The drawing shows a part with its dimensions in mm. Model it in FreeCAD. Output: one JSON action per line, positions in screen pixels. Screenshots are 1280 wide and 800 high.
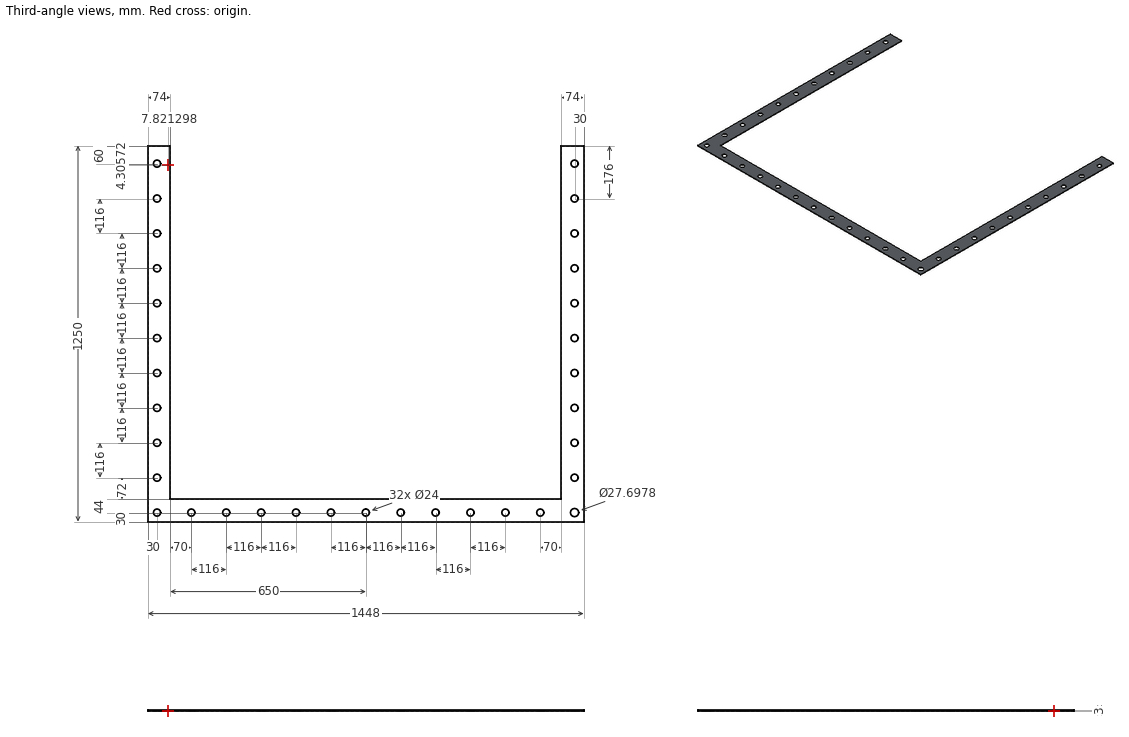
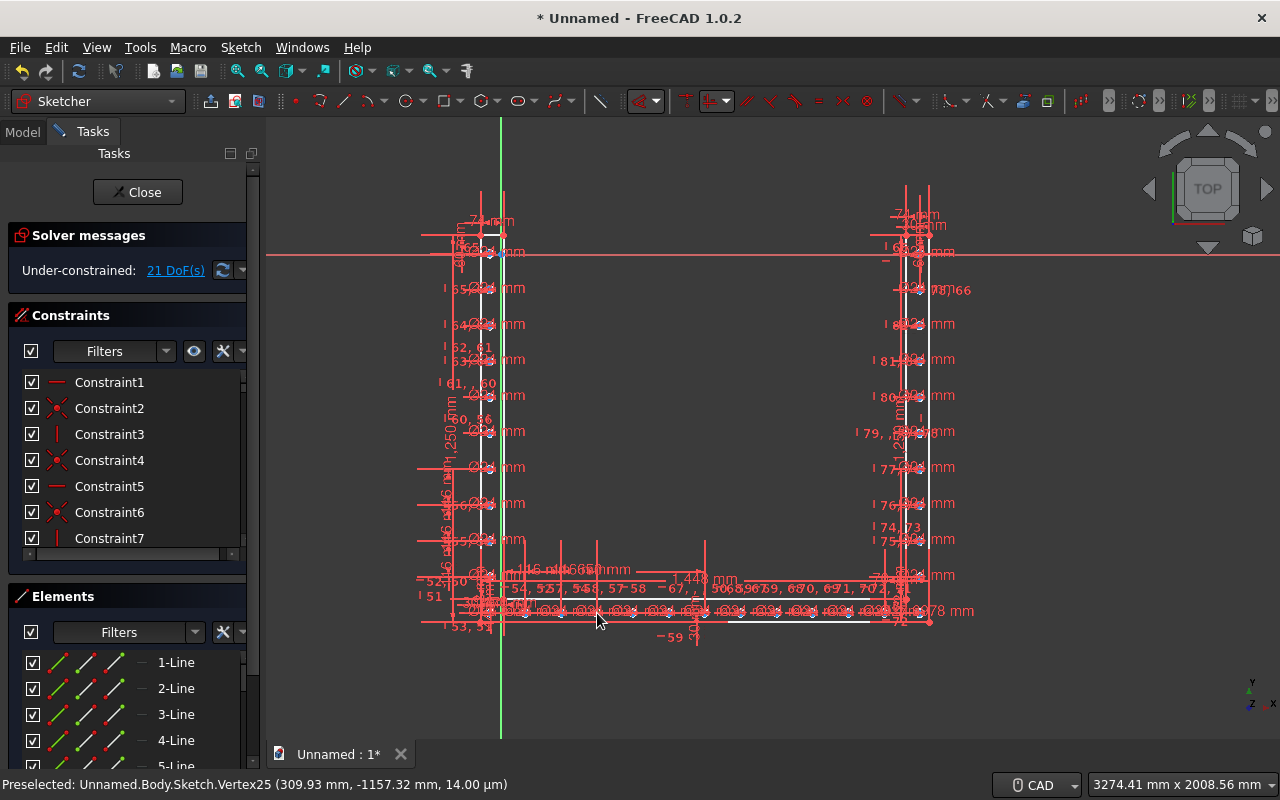
{"action": "left_click", "coordinate": [633, 613]}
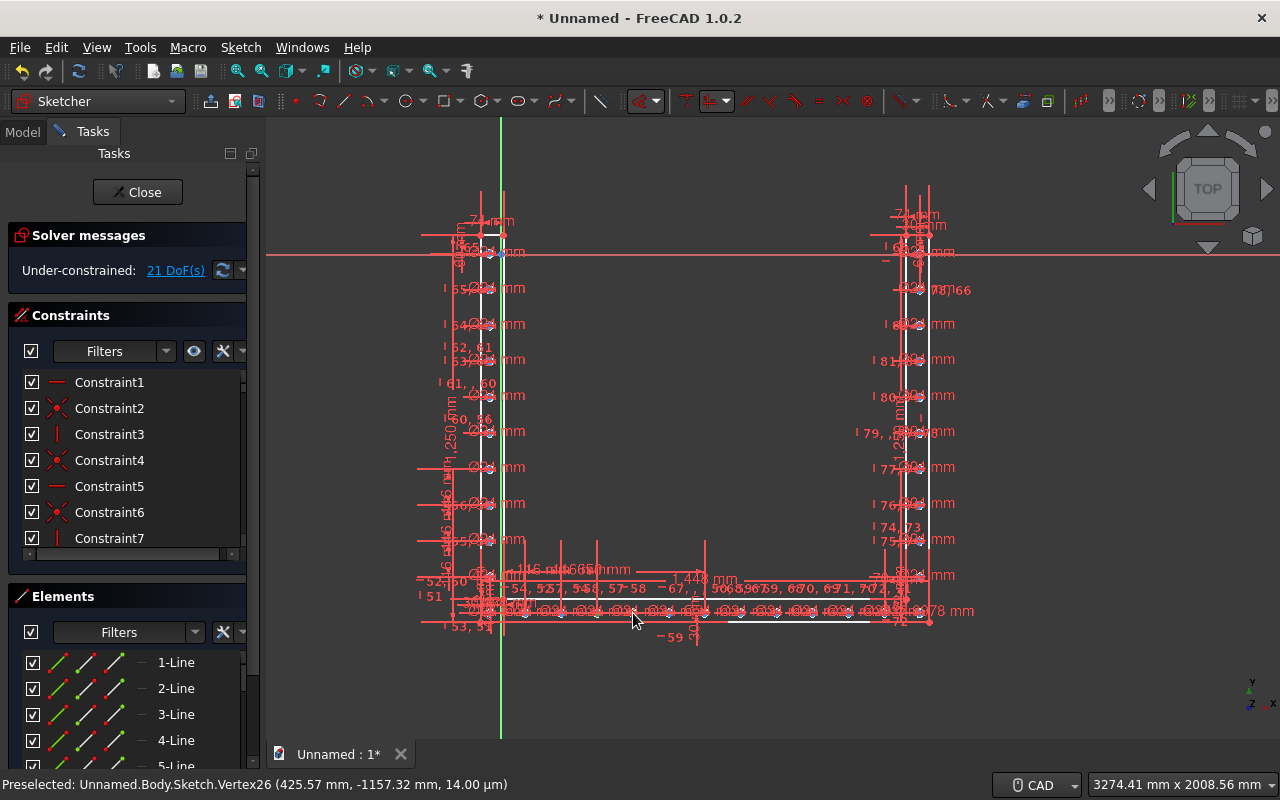
{"action": "key", "text": "l"}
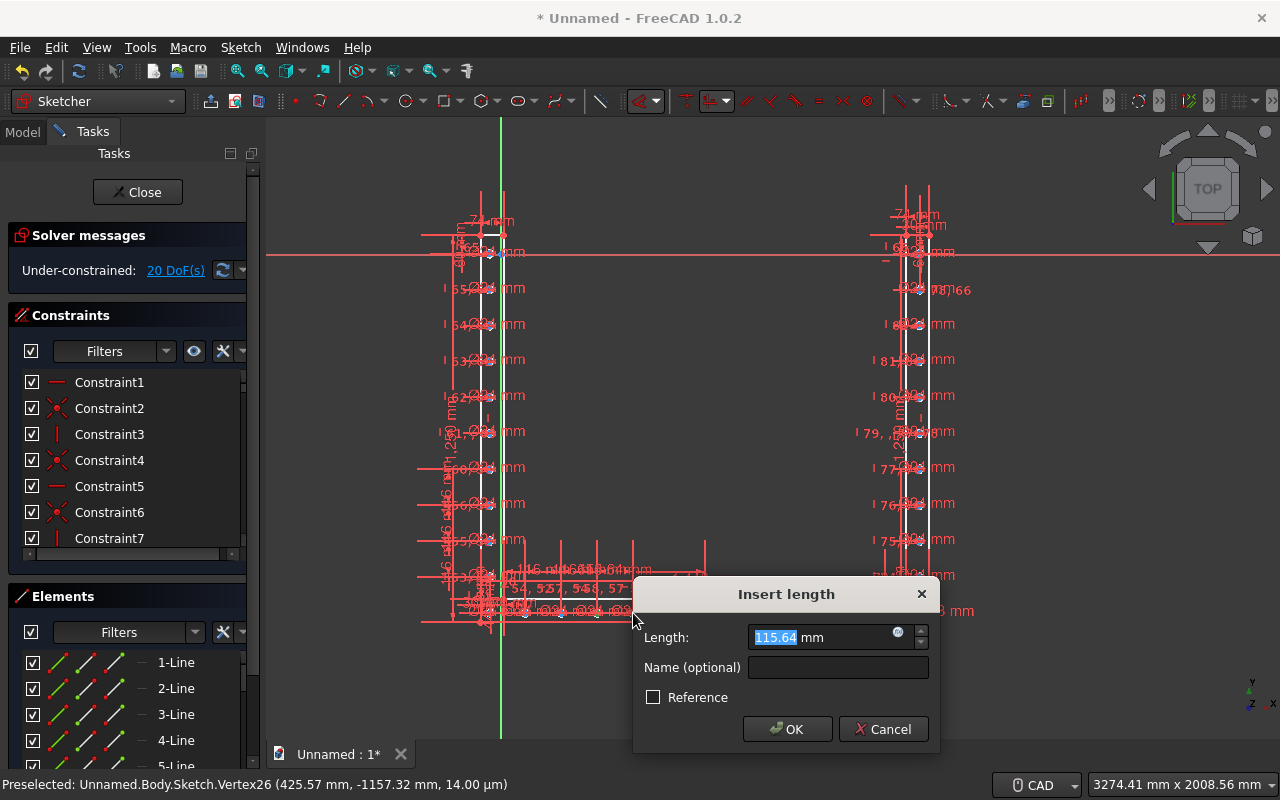
{"action": "type", "text": "116"}
{"action": "key", "text": "Return"}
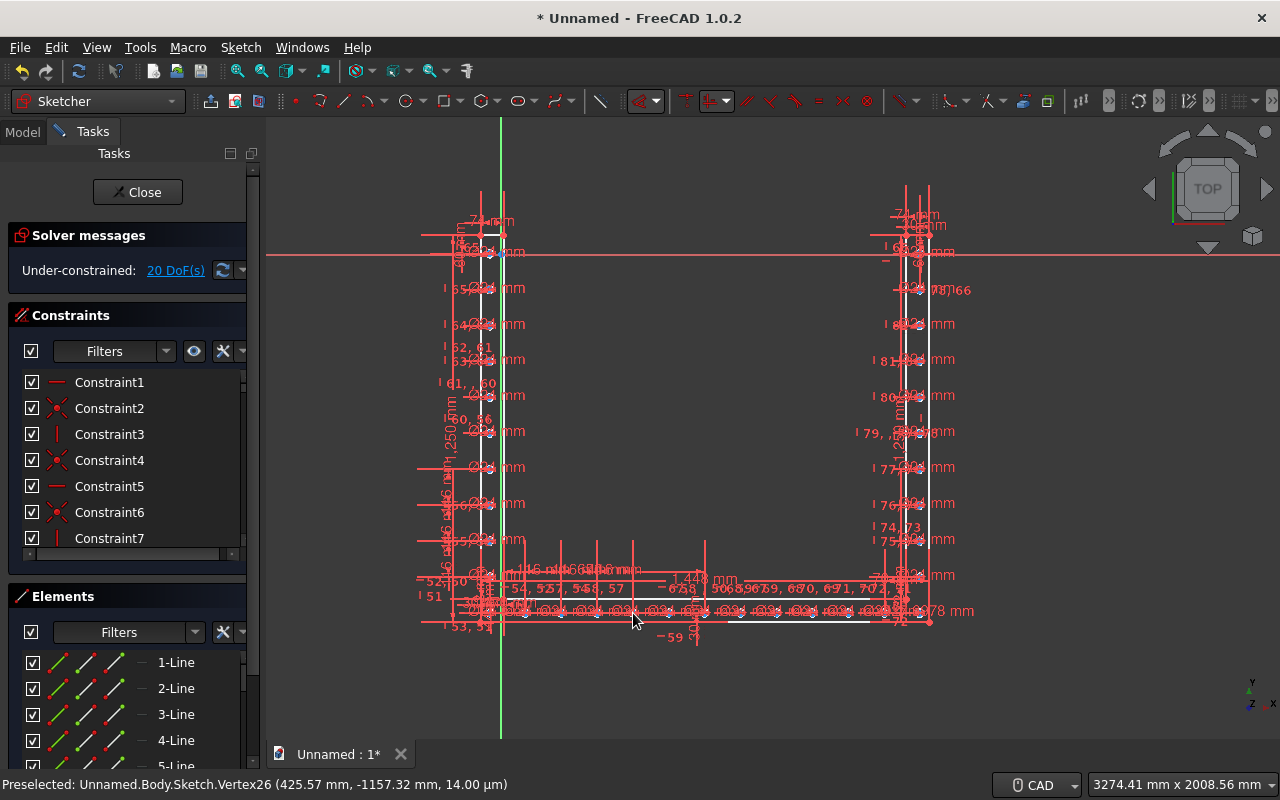
{"action": "left_click", "coordinate": [705, 613]}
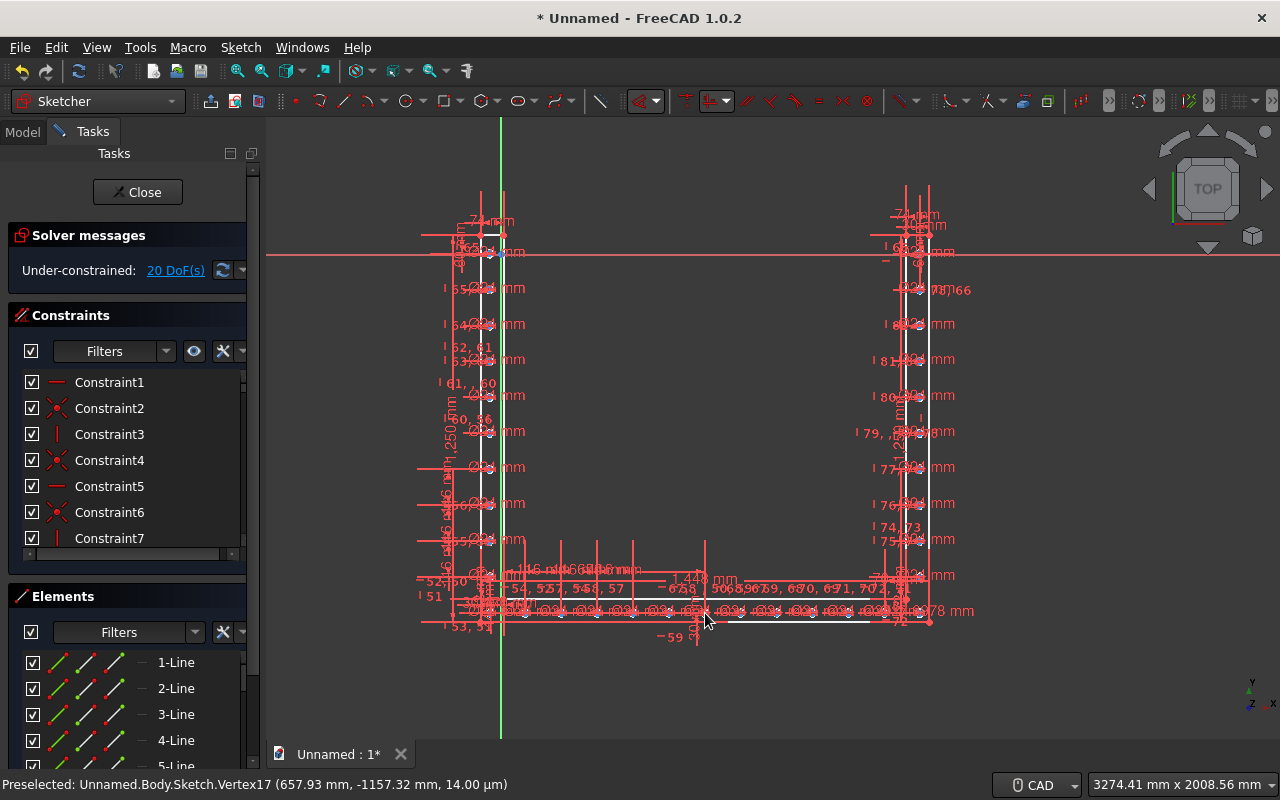
{"action": "left_click", "coordinate": [669, 613]}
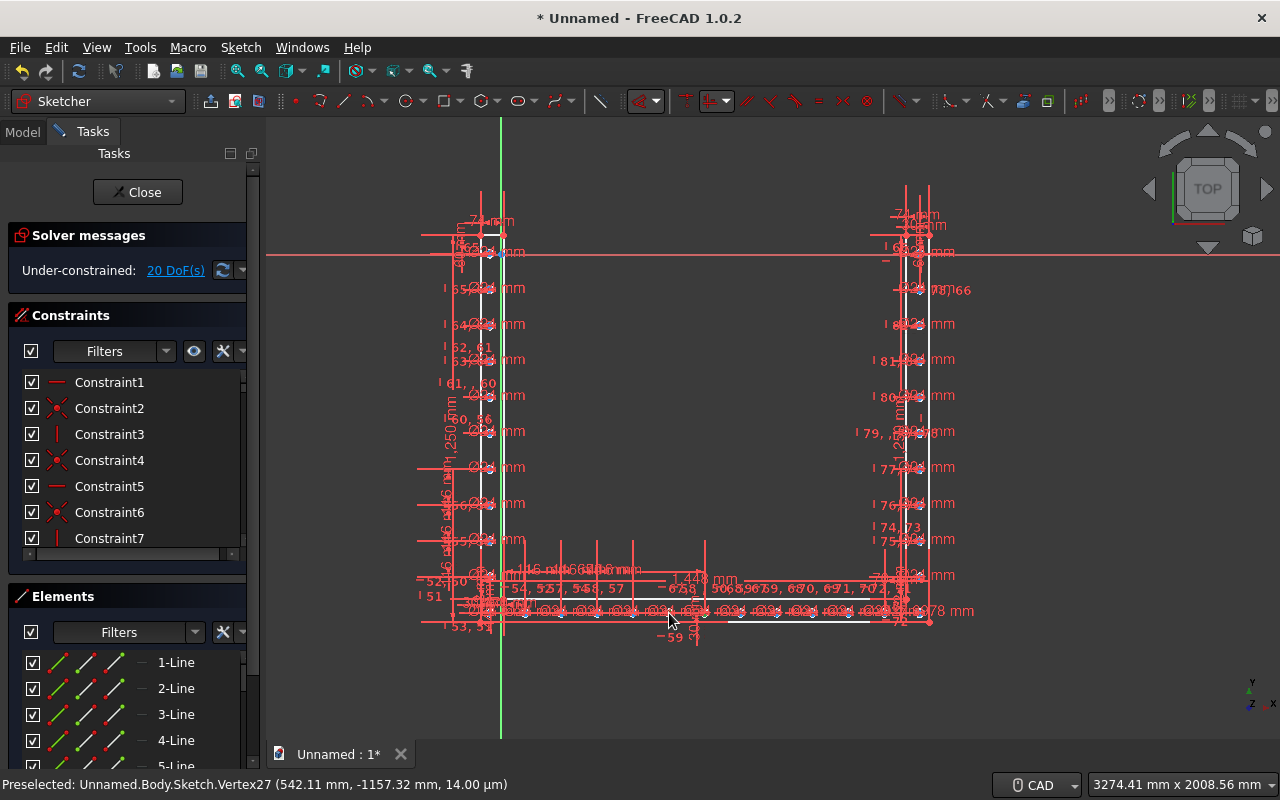
{"action": "left_click", "coordinate": [658, 102]}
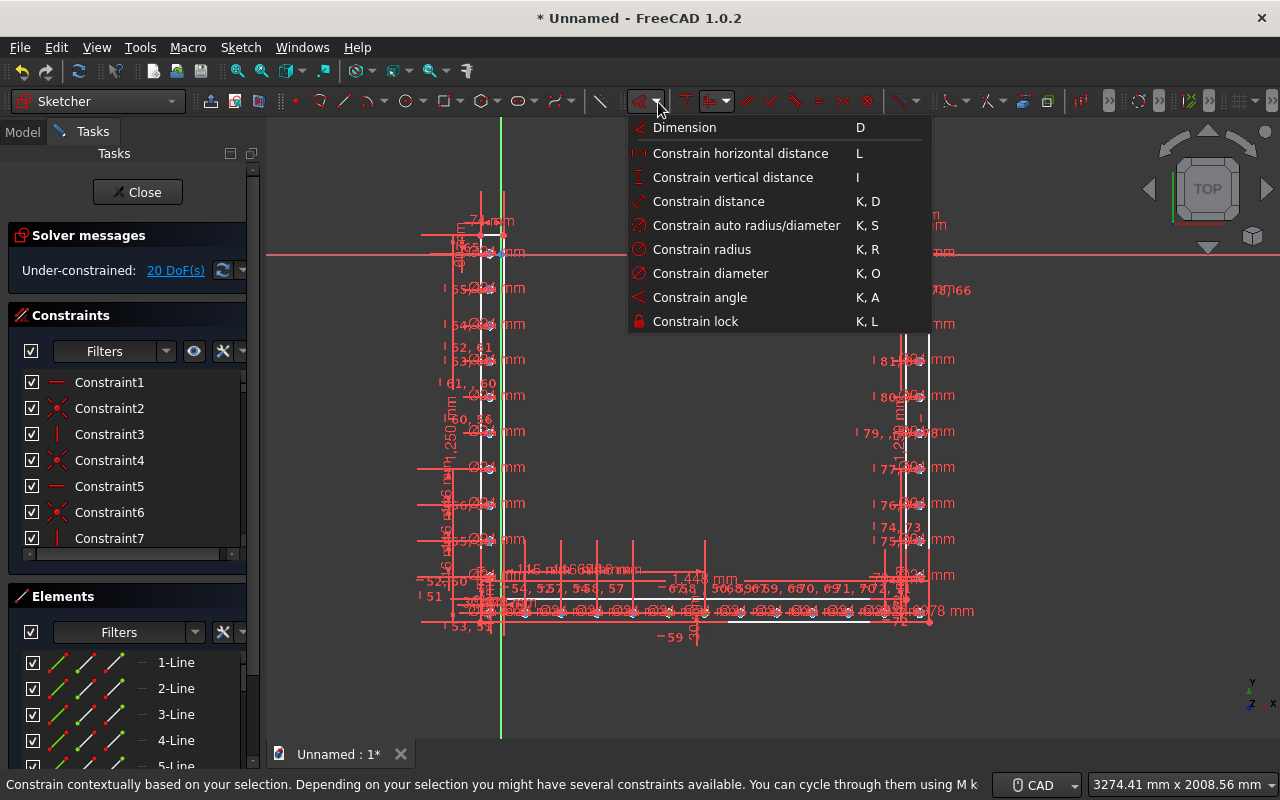
{"action": "left_click", "coordinate": [780, 153]}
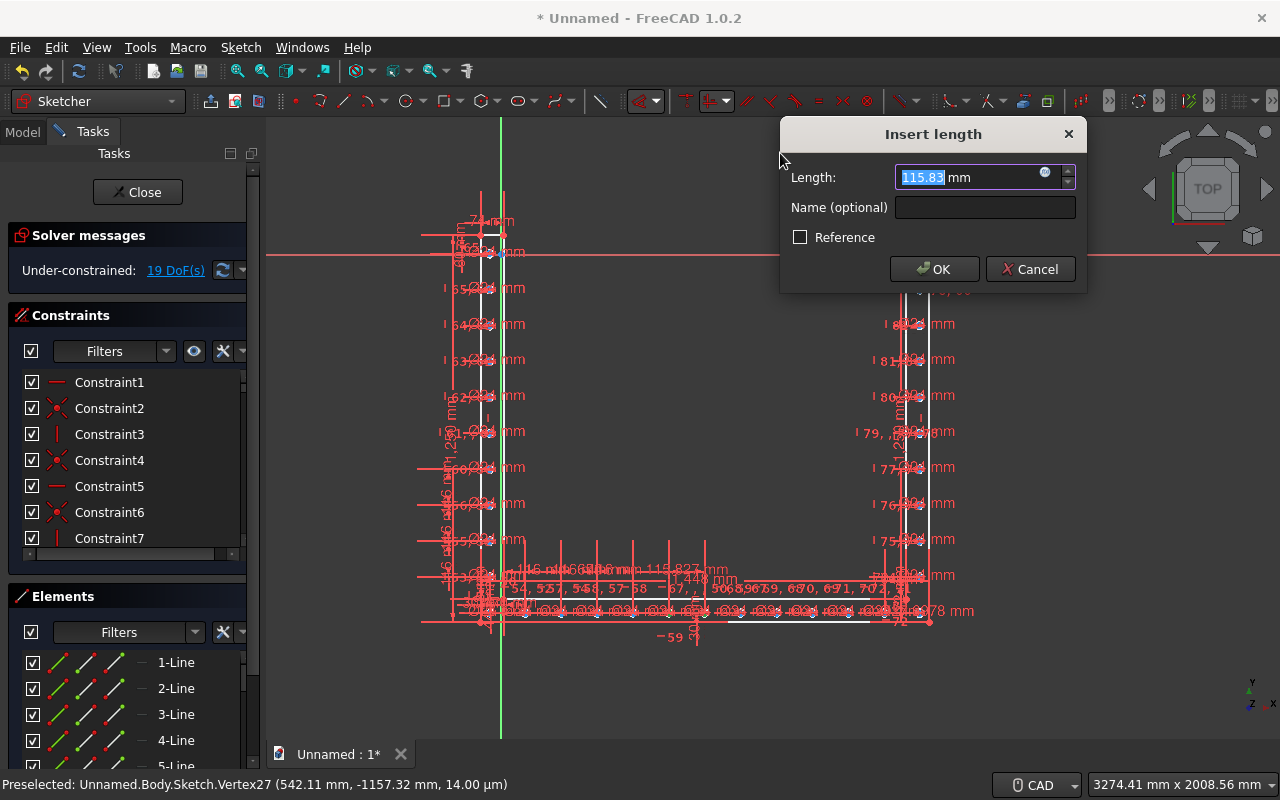
{"action": "type", "text": "116"}
{"action": "key", "text": "Return"}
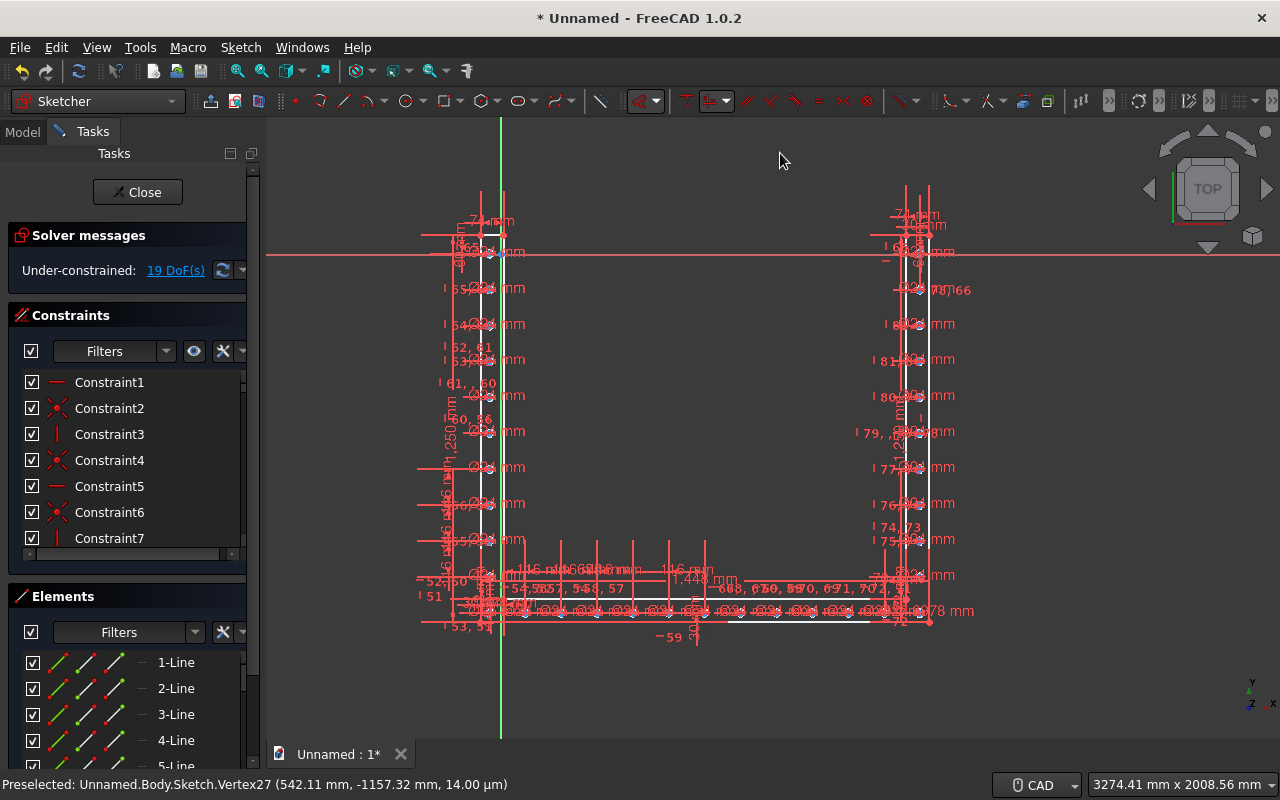
{"action": "left_click", "coordinate": [490, 469]}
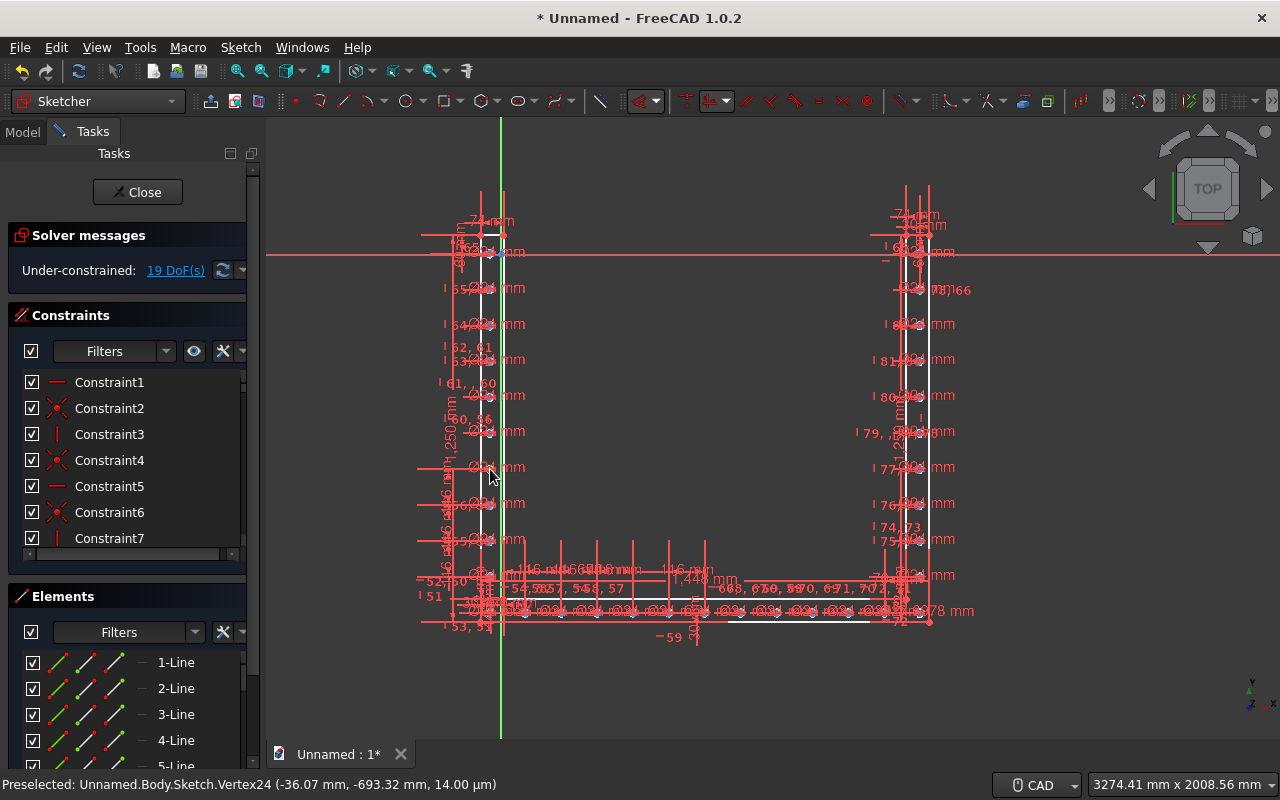
{"action": "left_click", "coordinate": [490, 433]}